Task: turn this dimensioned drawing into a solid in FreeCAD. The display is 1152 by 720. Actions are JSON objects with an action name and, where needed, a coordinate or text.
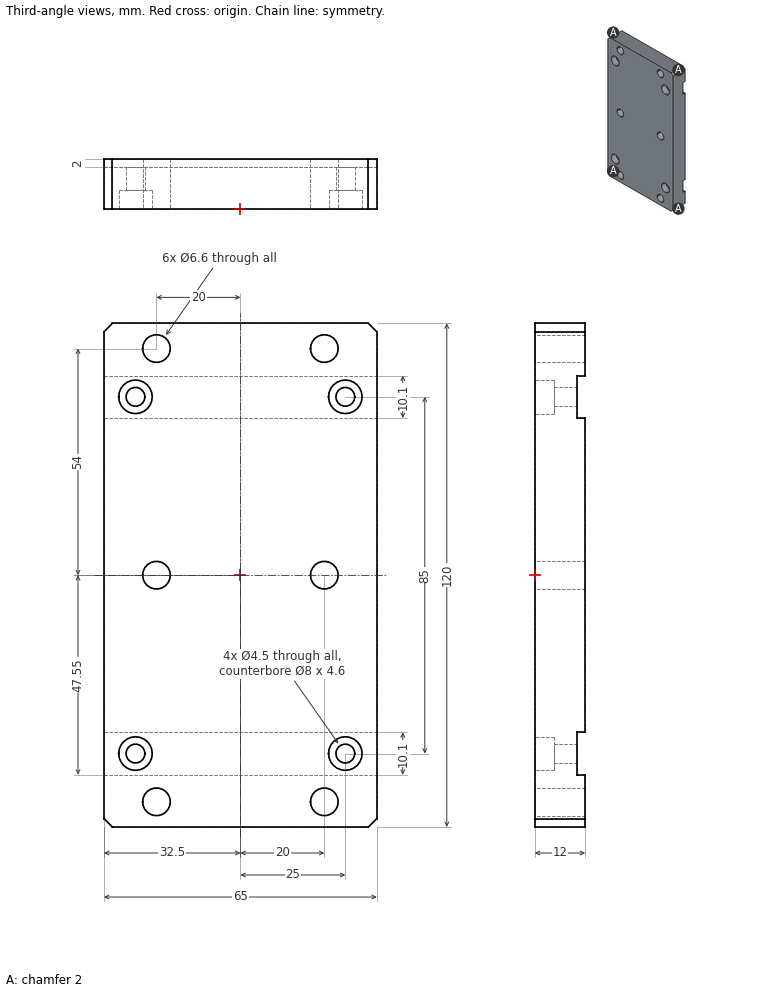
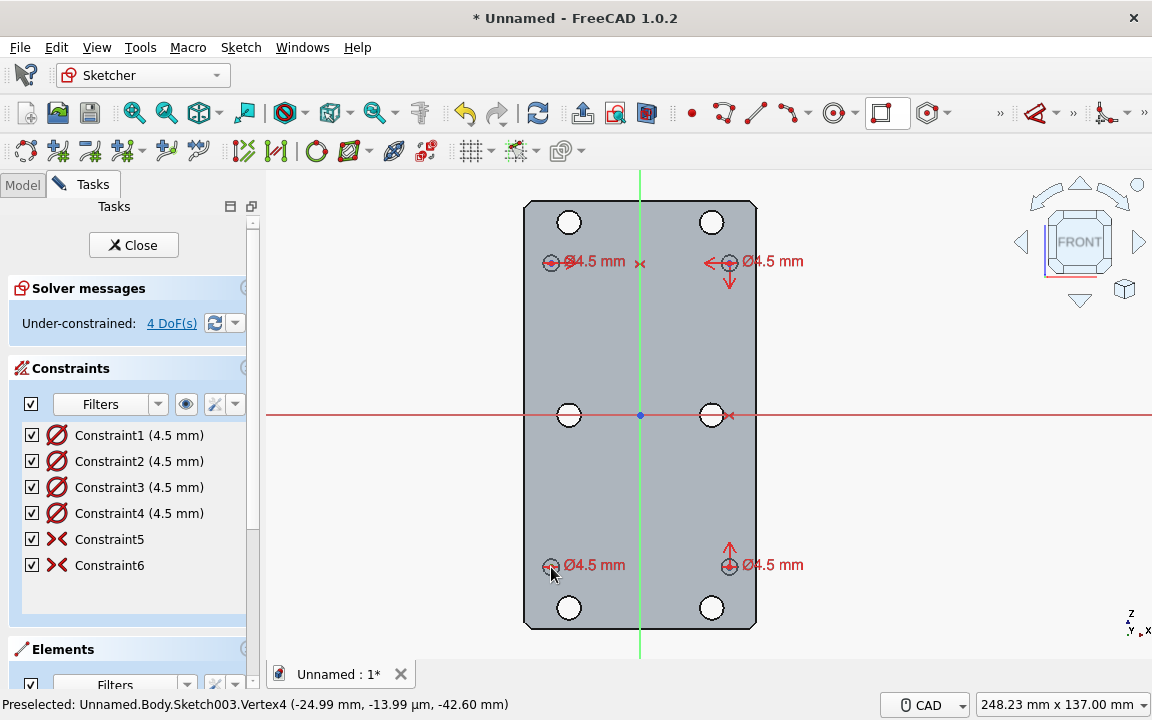
{"action": "left_click", "coordinate": [640, 600]}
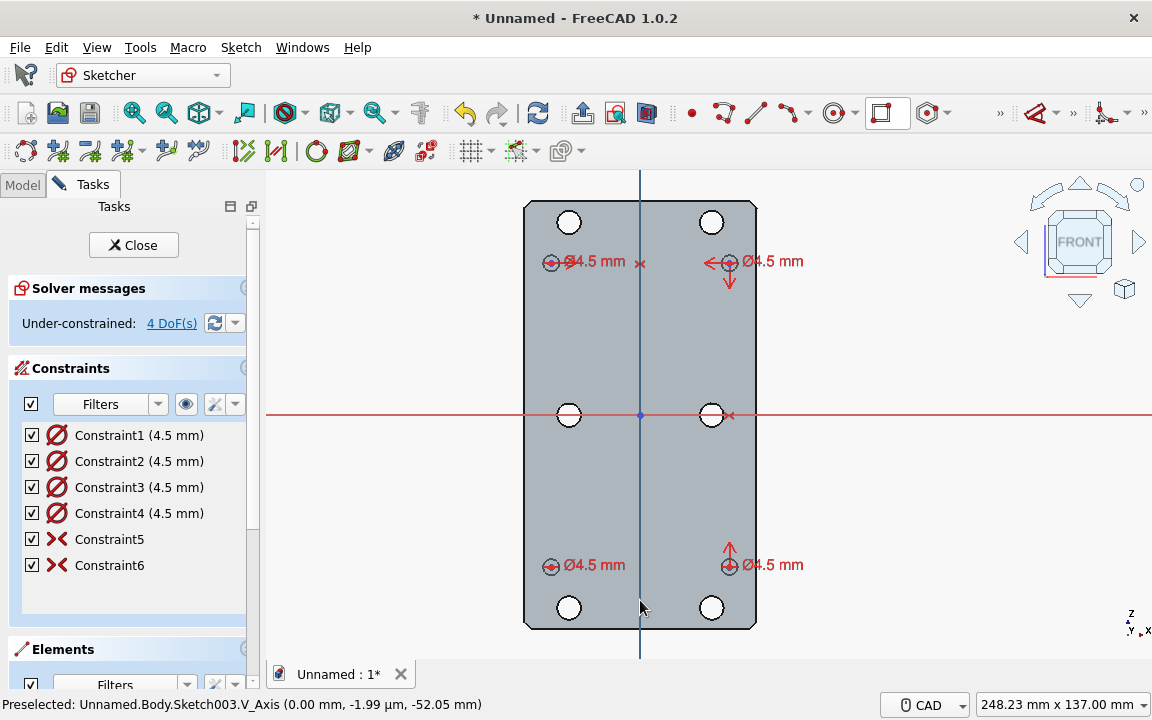
{"action": "key", "text": "s"}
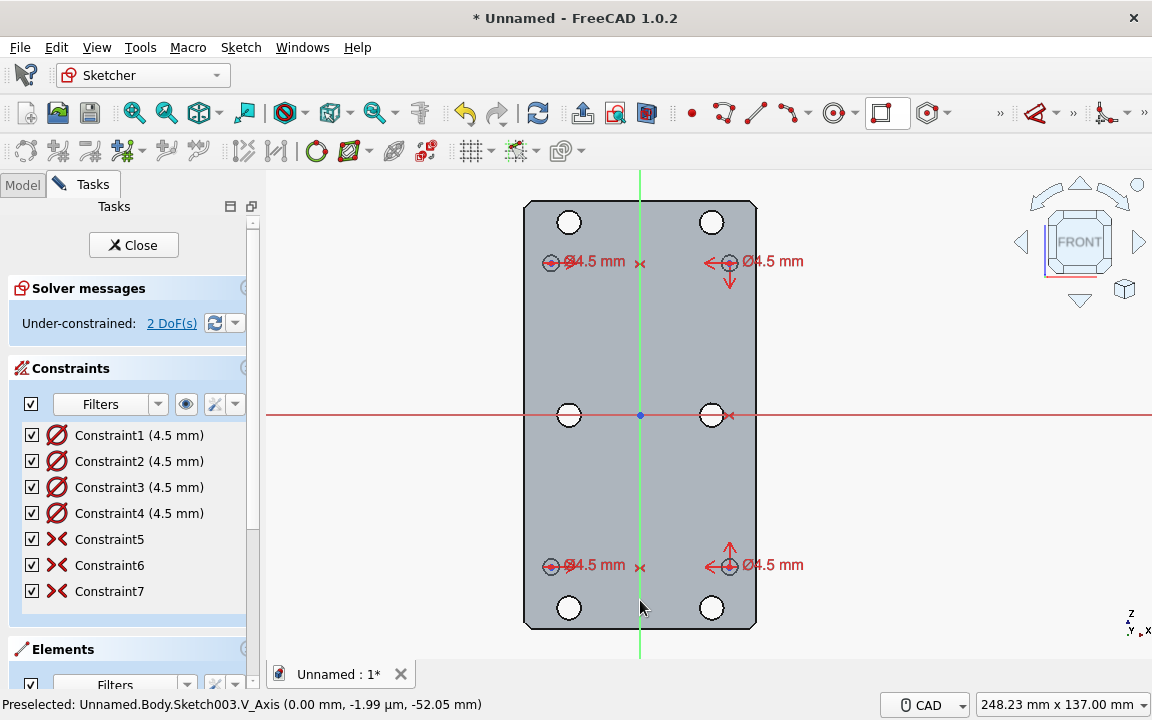
{"action": "key", "text": "d"}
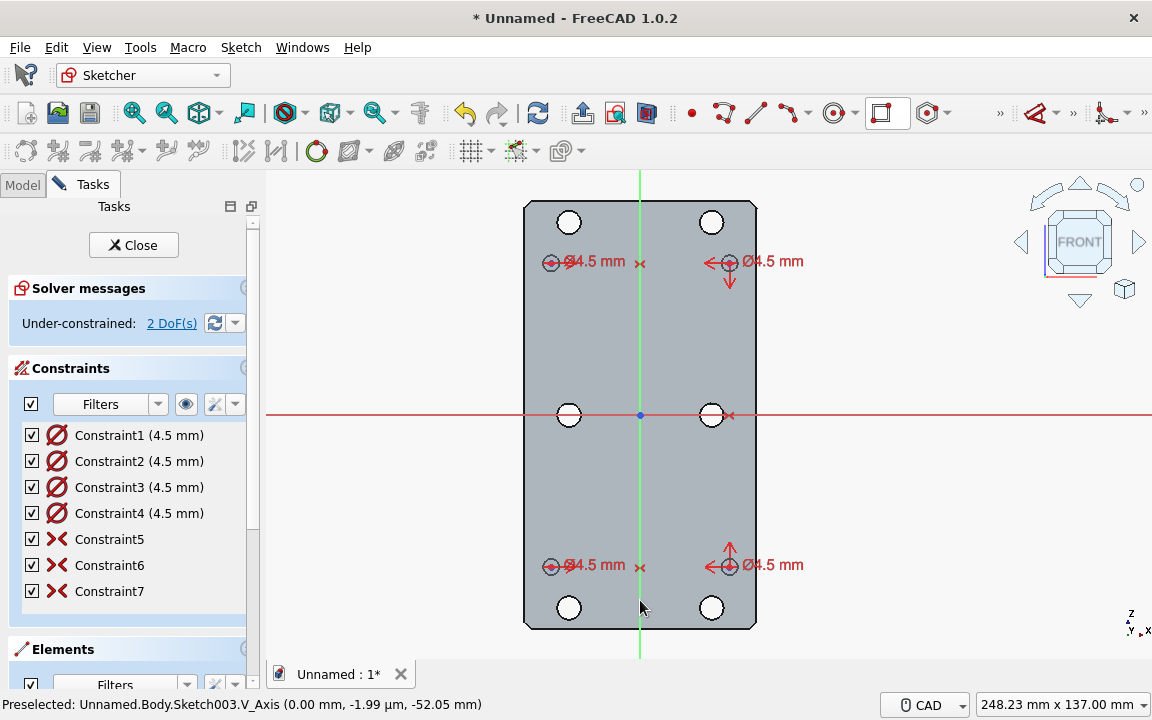
{"action": "left_click", "coordinate": [730, 567]}
{"action": "left_click", "coordinate": [685, 601]}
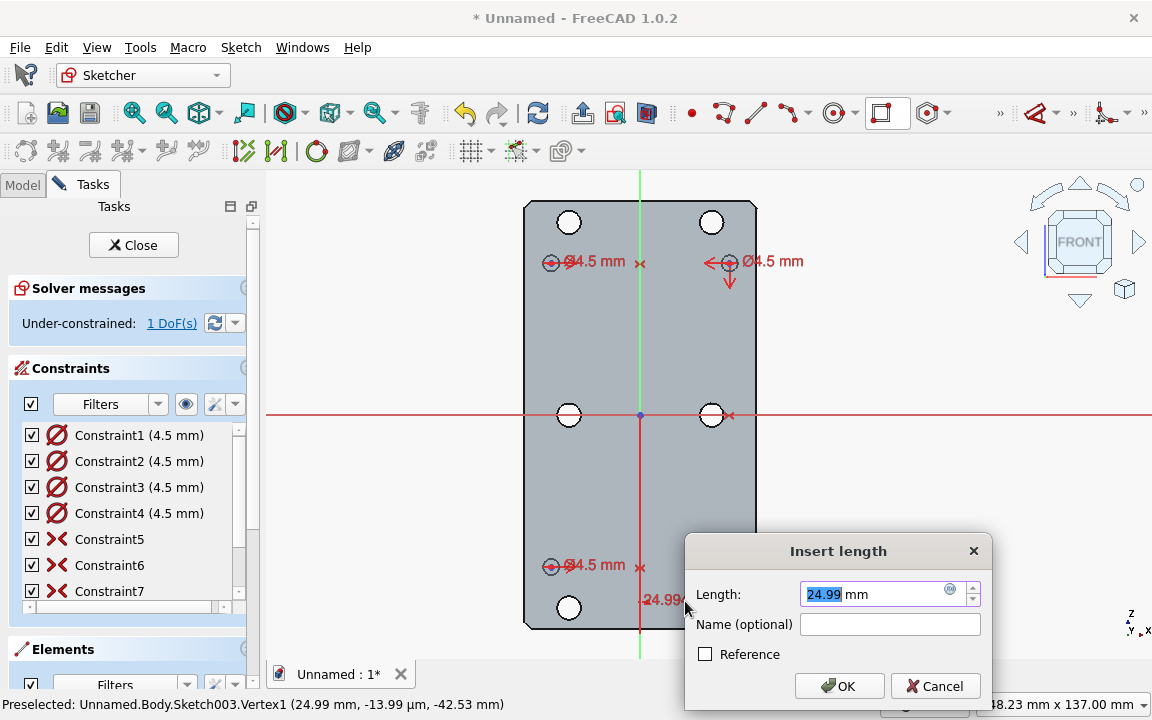
{"action": "type", "text": "25"}
{"action": "key", "text": "Return"}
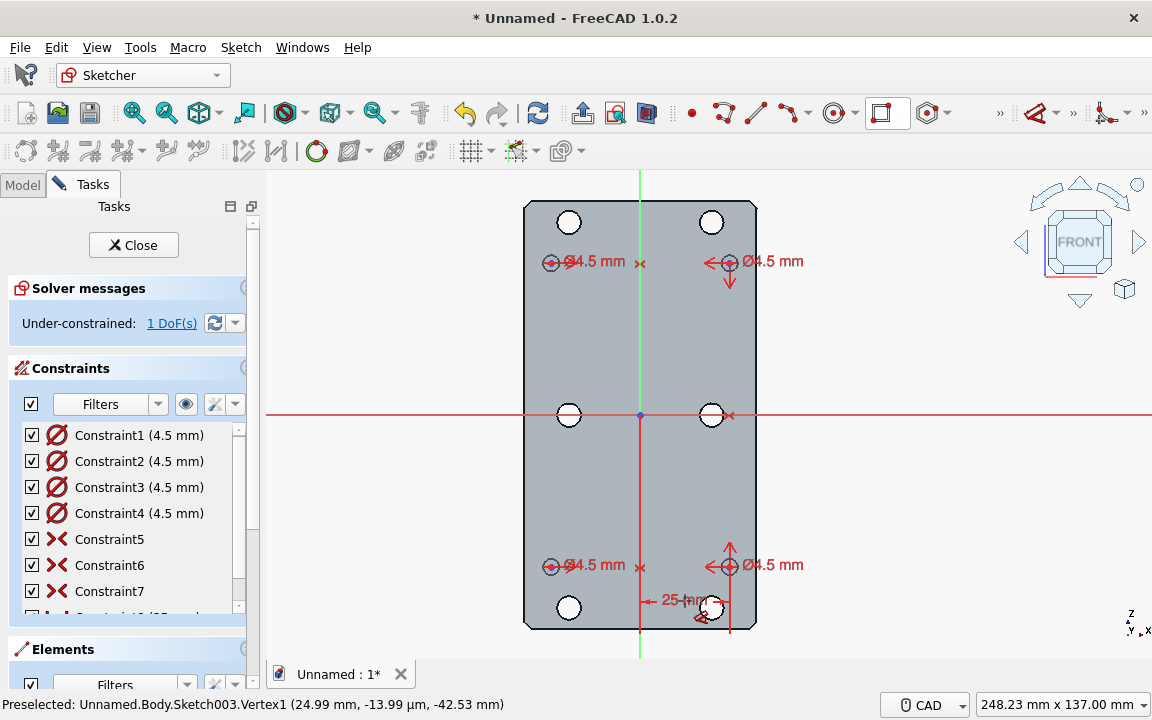
{"action": "left_click", "coordinate": [730, 567]}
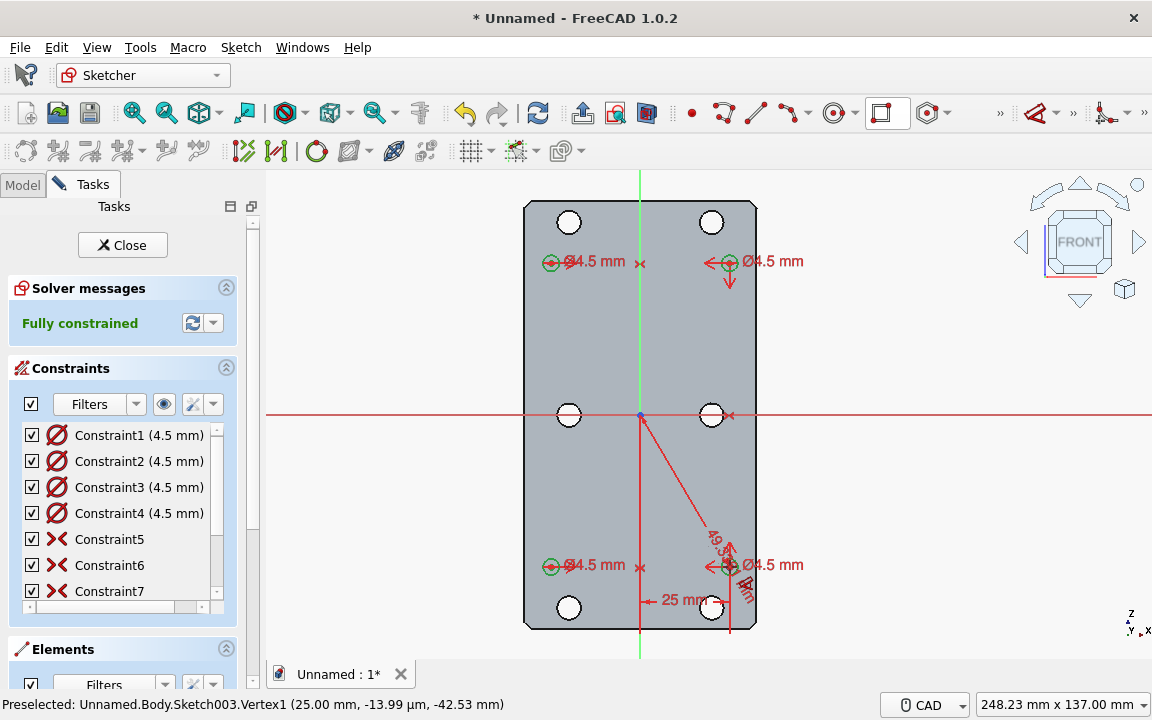
{"action": "left_click", "coordinate": [730, 263]}
{"action": "left_click", "coordinate": [764, 345]}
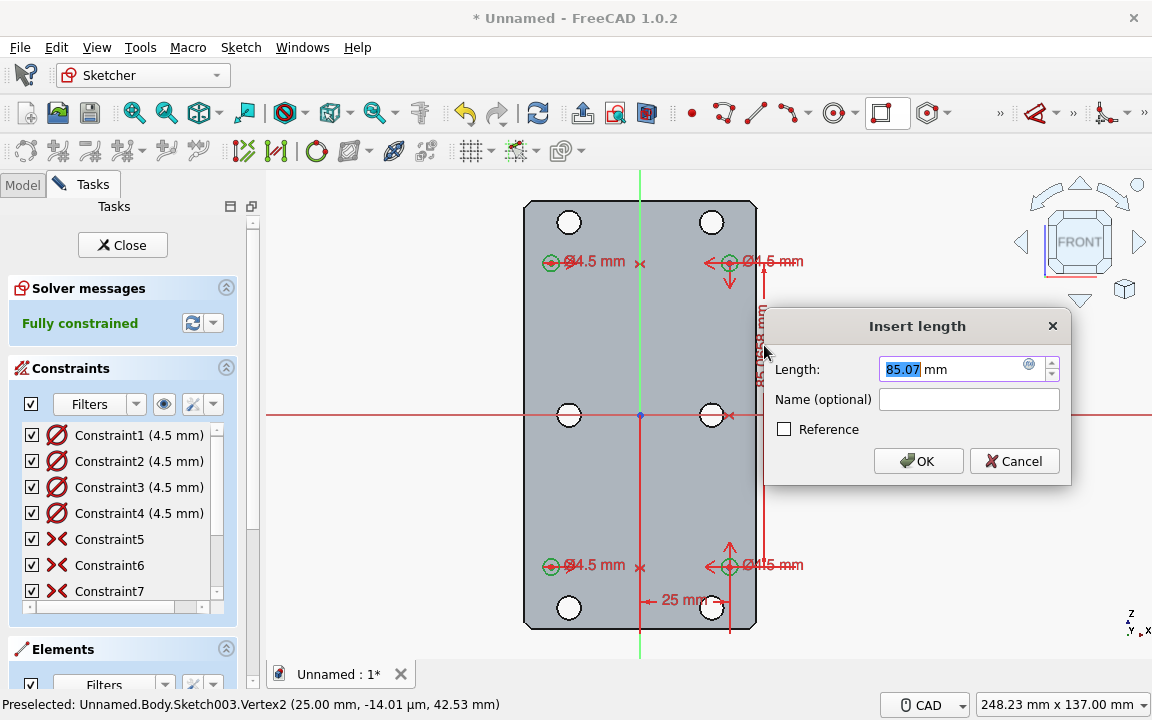
{"action": "type", "text": "85"}
{"action": "key", "text": "Return"}
{"action": "key", "text": "Escape"}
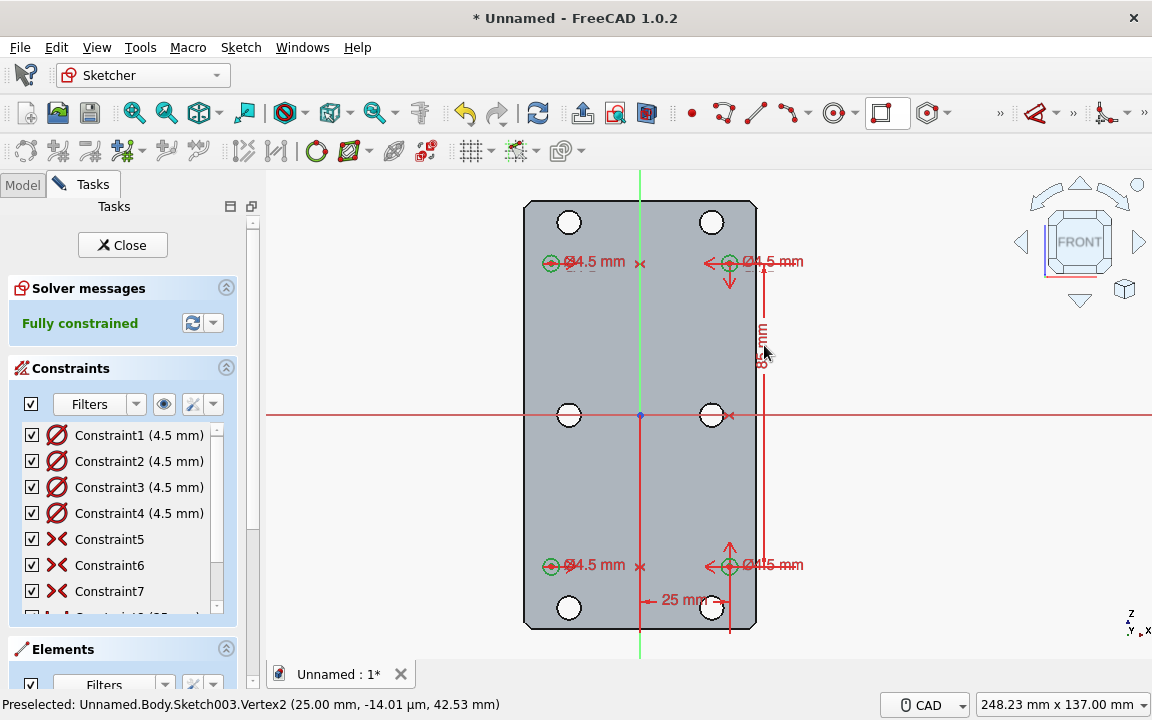
{"action": "left_click", "coordinate": [123, 245]}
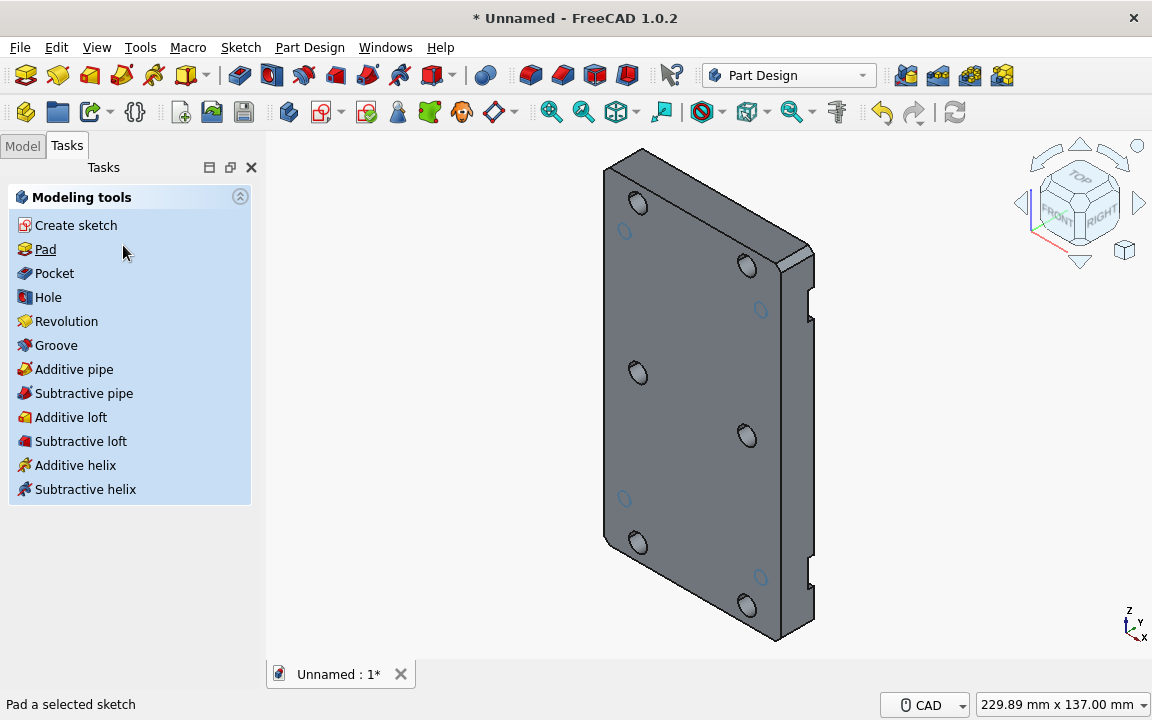
{"action": "left_click", "coordinate": [272, 76]}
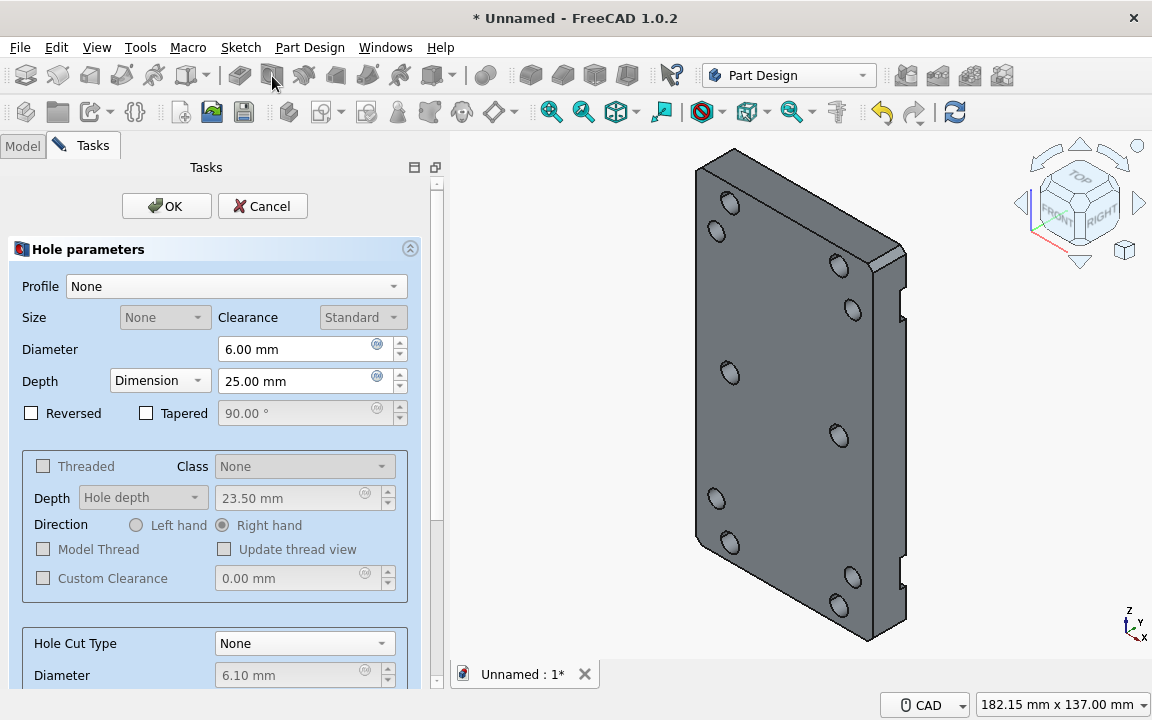
{"action": "triple_click", "coordinate": [305, 349]}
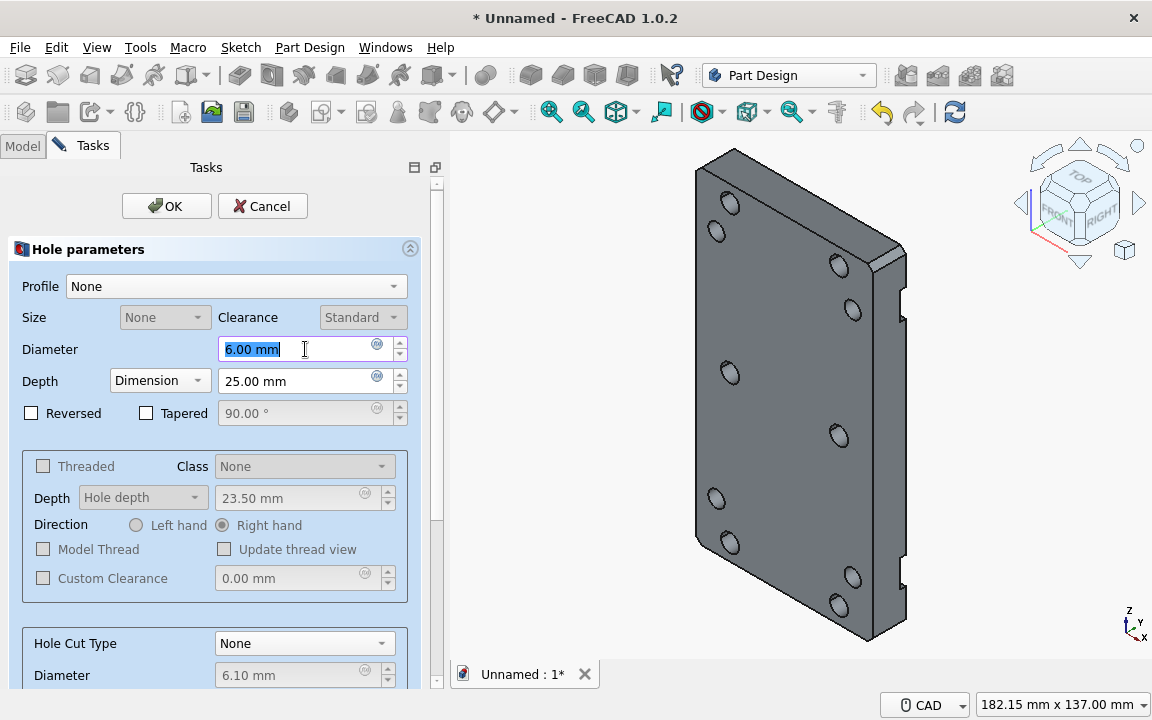
{"action": "type", "text": "4.5"}
{"action": "key", "text": "Tab"}